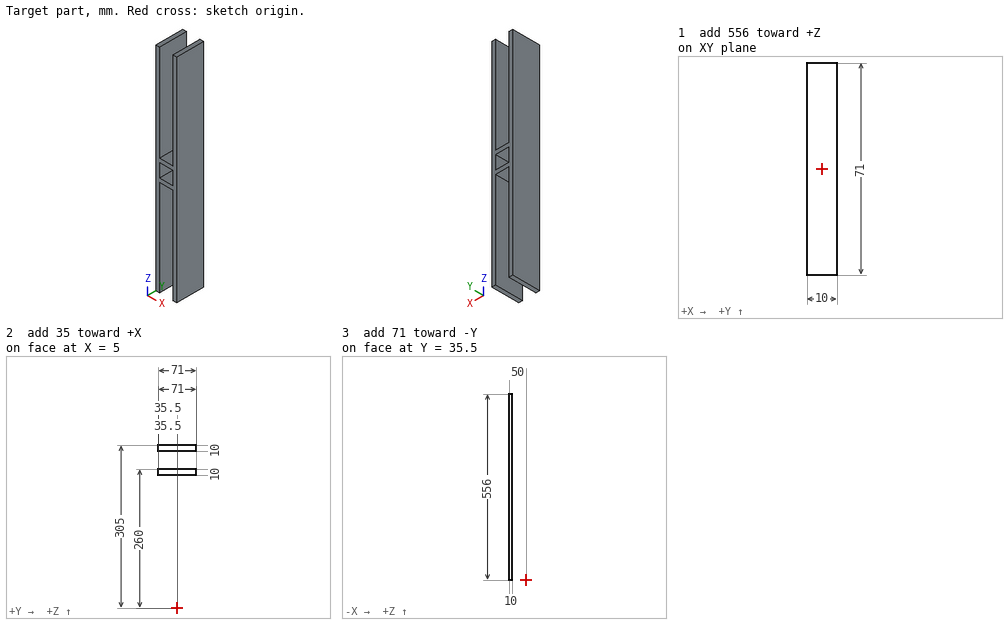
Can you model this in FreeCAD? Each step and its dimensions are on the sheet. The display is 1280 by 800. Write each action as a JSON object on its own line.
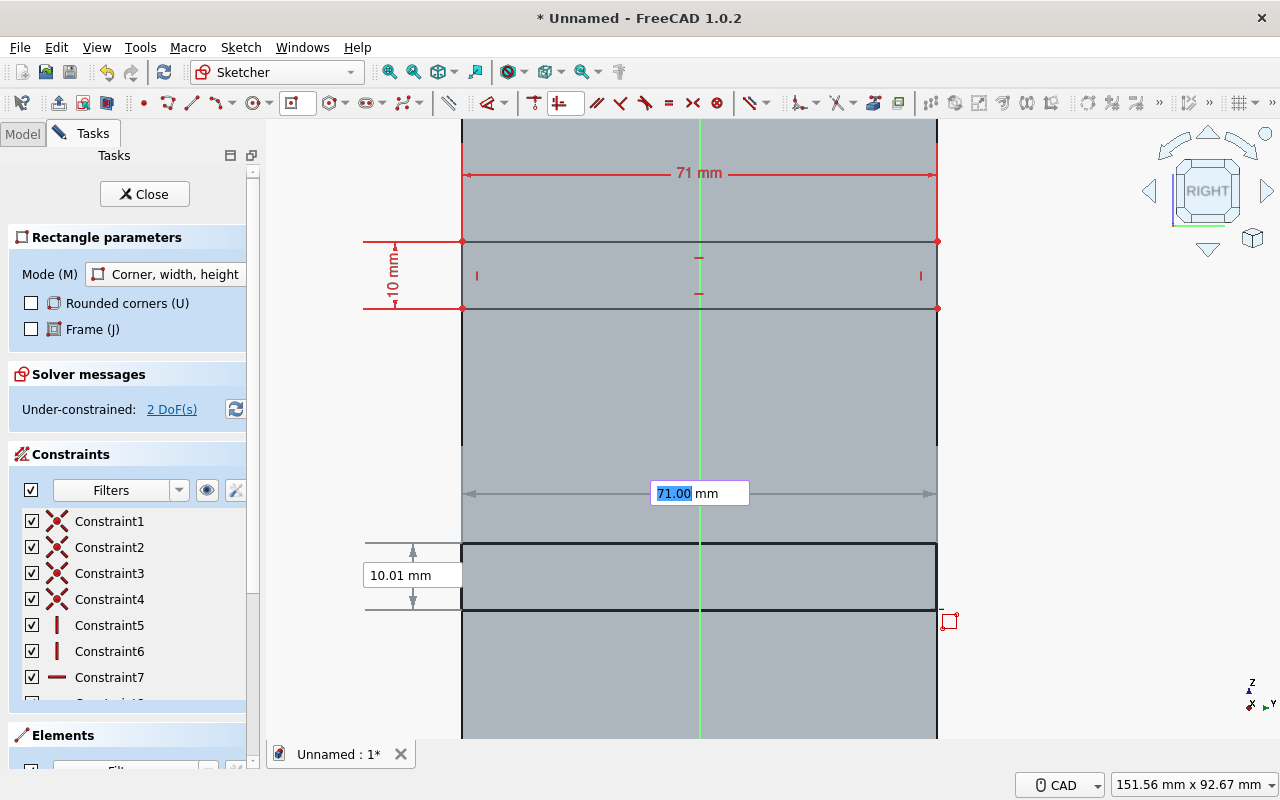
{"action": "type", "text": "71"}
{"action": "key", "text": "Tab"}
{"action": "type", "text": "10"}
{"action": "key", "text": "Return"}
{"action": "key", "text": "Escape"}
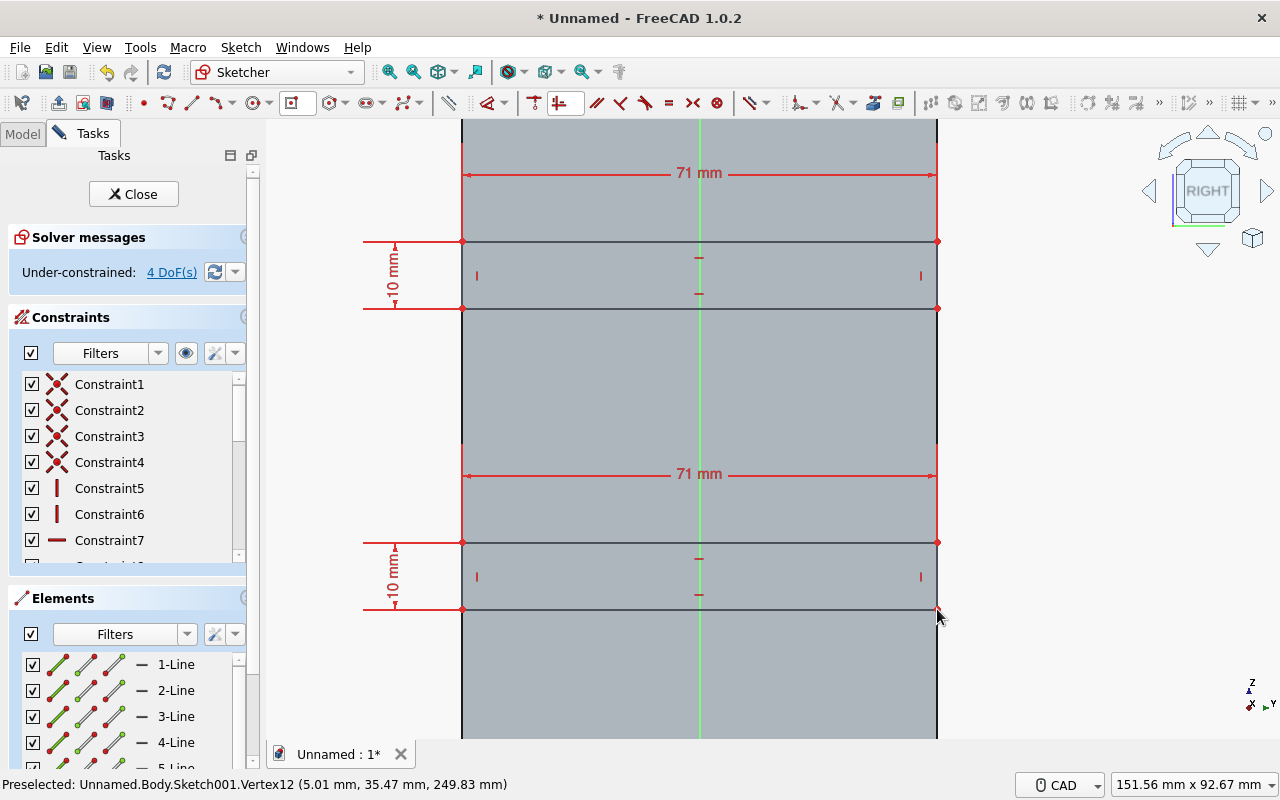
{"action": "left_click", "coordinate": [462, 242]}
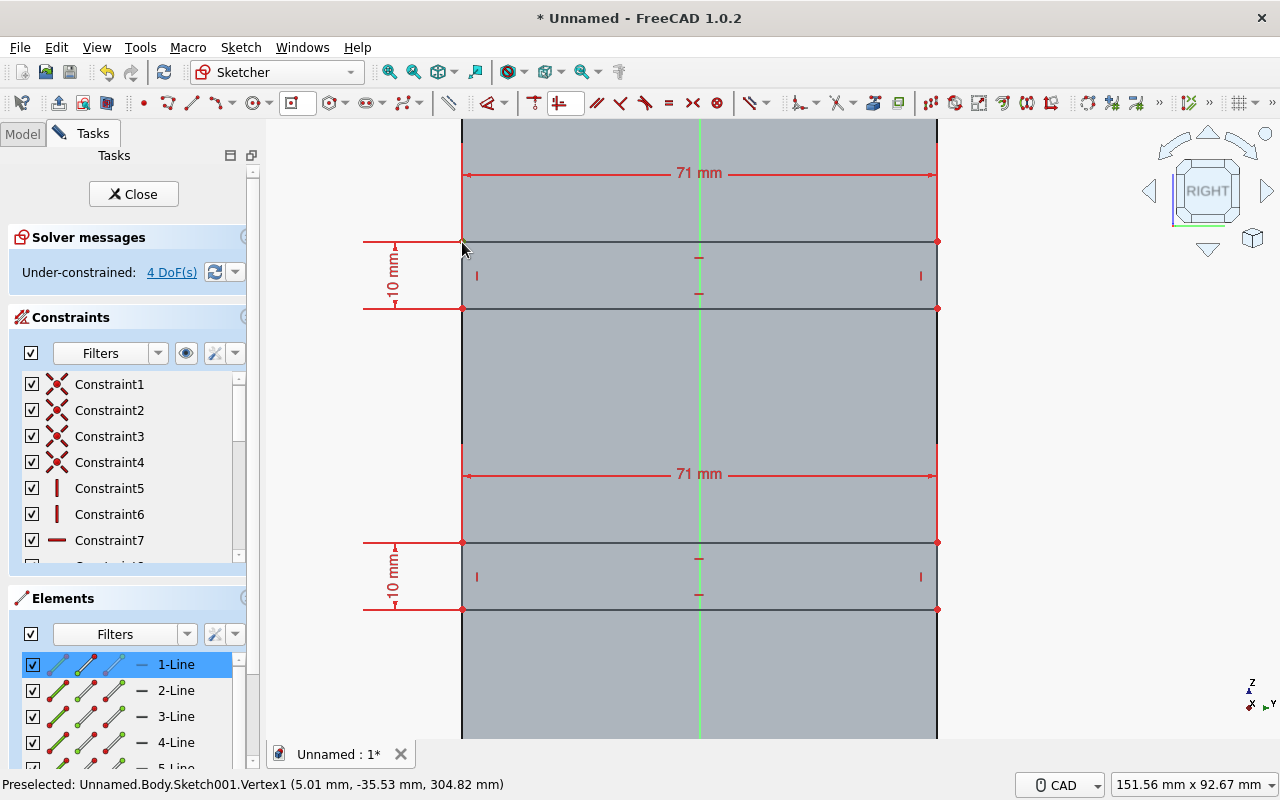
{"action": "left_click", "coordinate": [506, 104]}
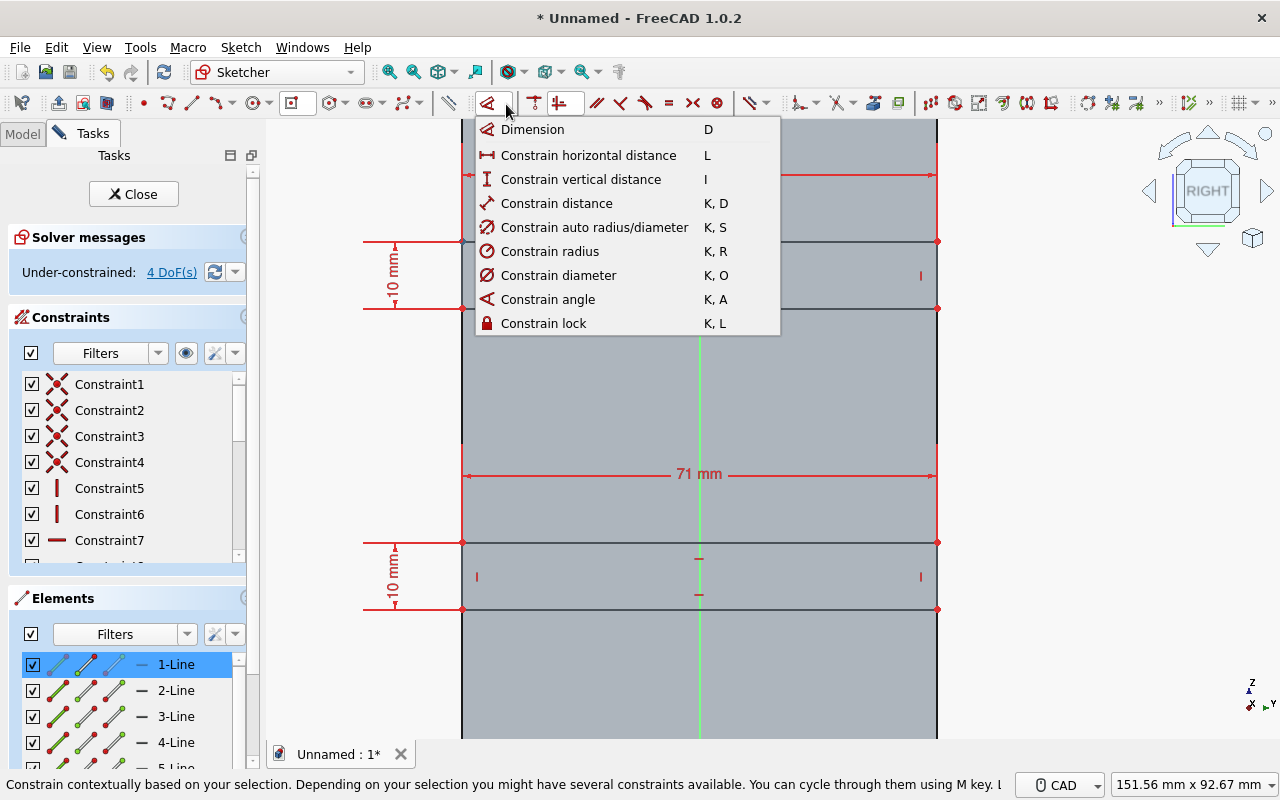
{"action": "left_click", "coordinate": [628, 179]}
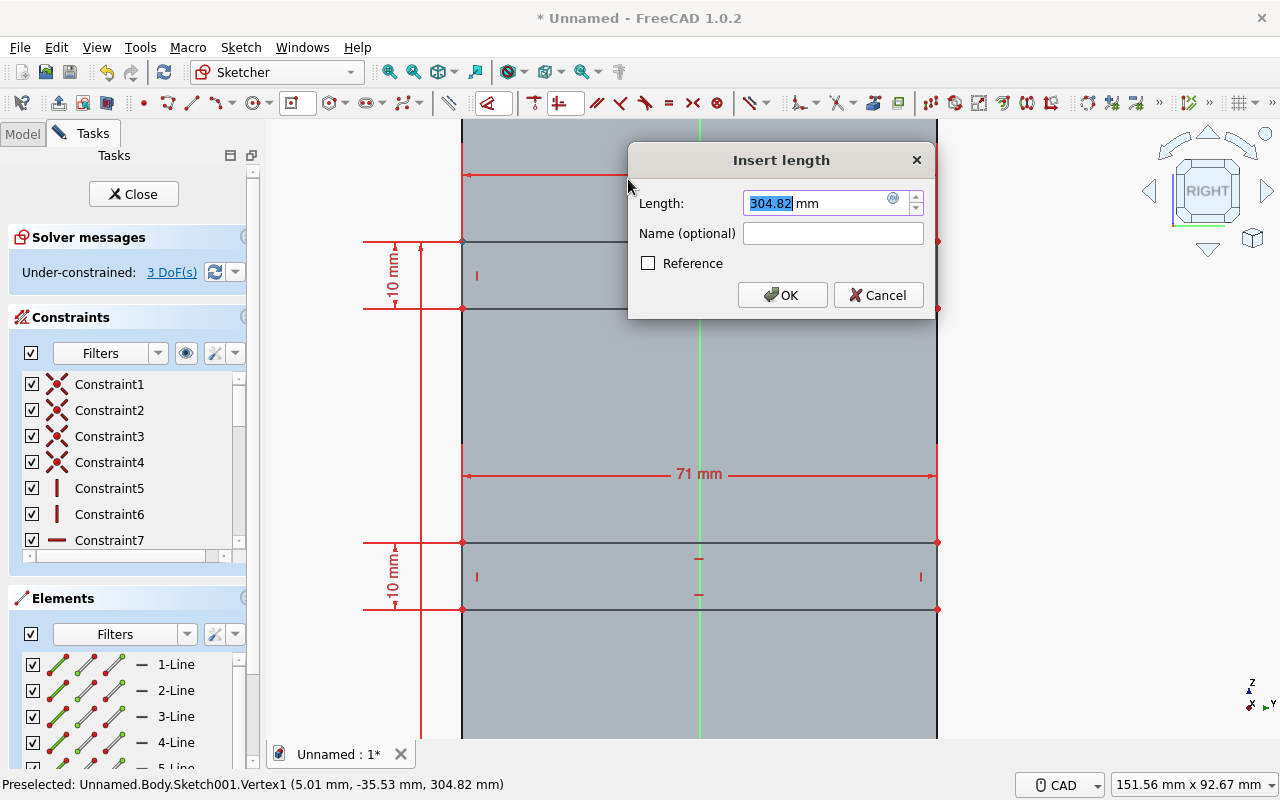
{"action": "type", "text": "305"}
{"action": "key", "text": "Return"}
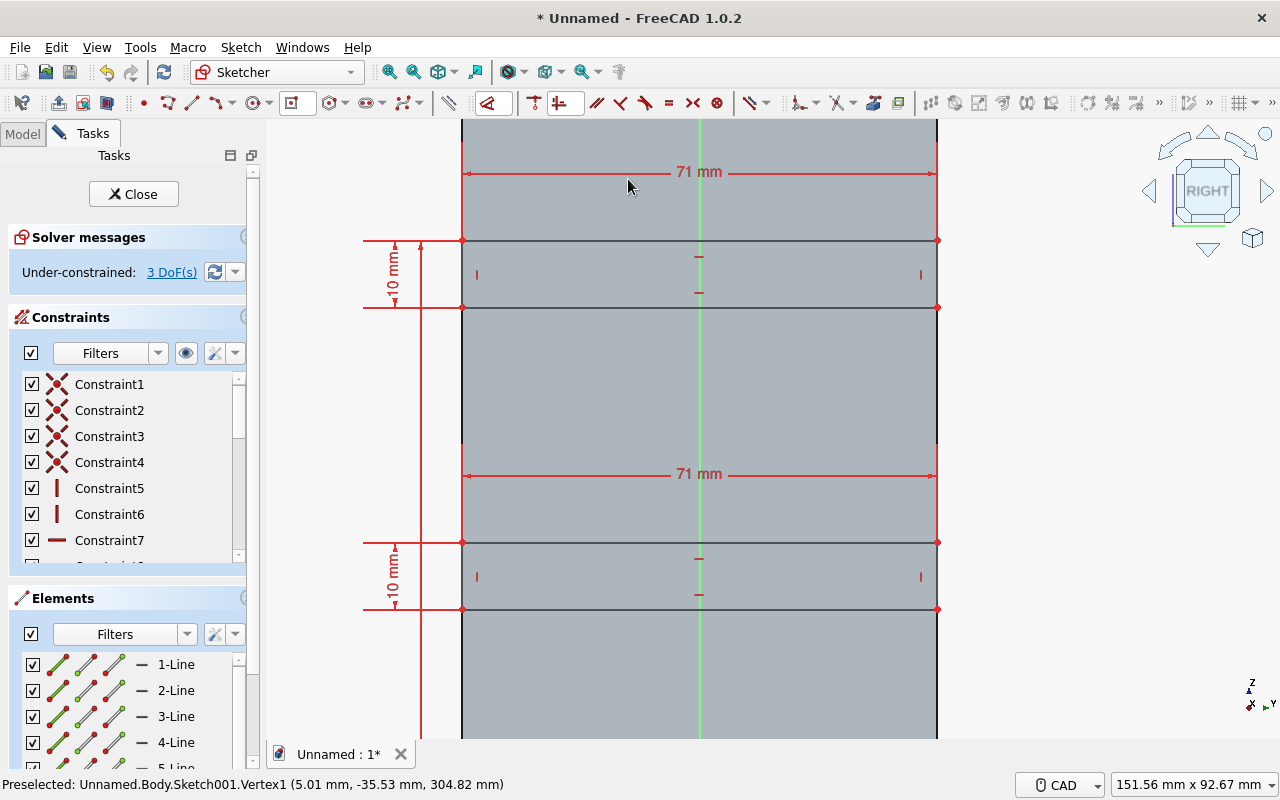
{"action": "left_click", "coordinate": [462, 543]}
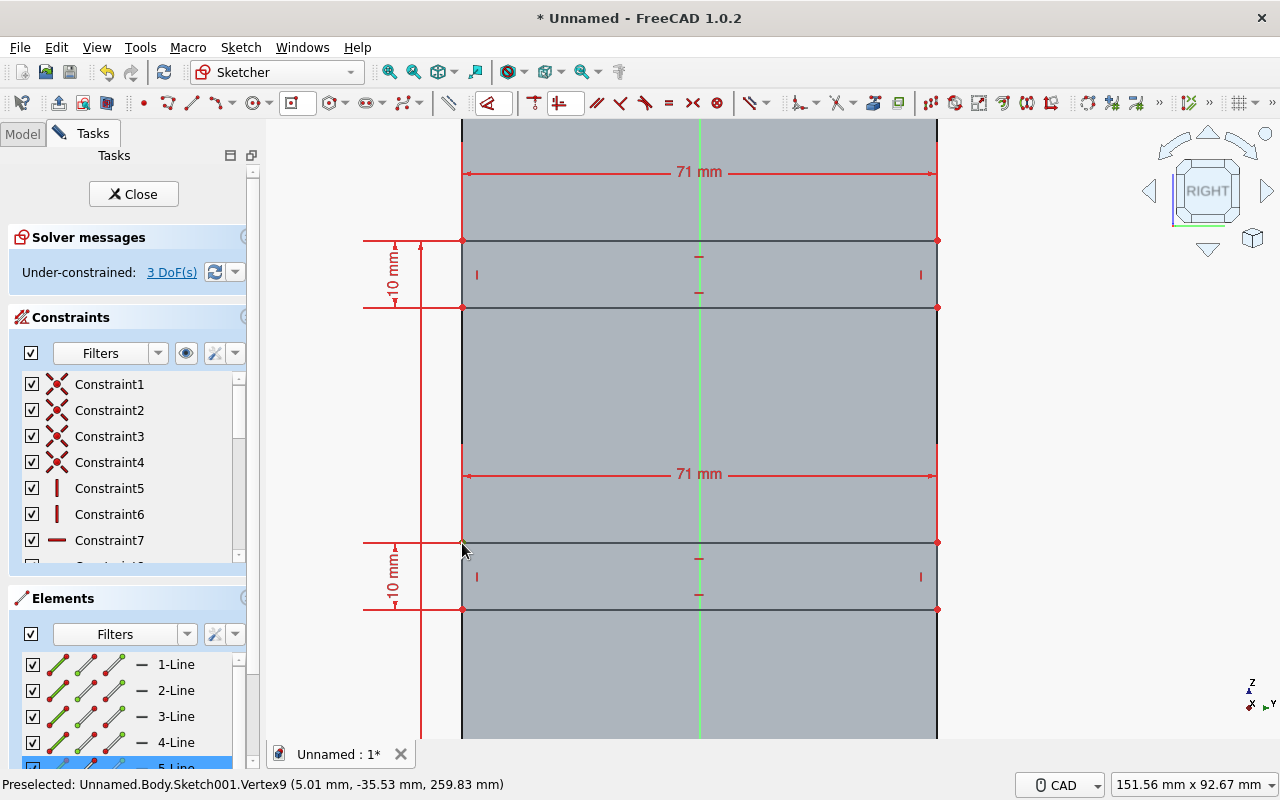
{"action": "left_click", "coordinate": [506, 104]}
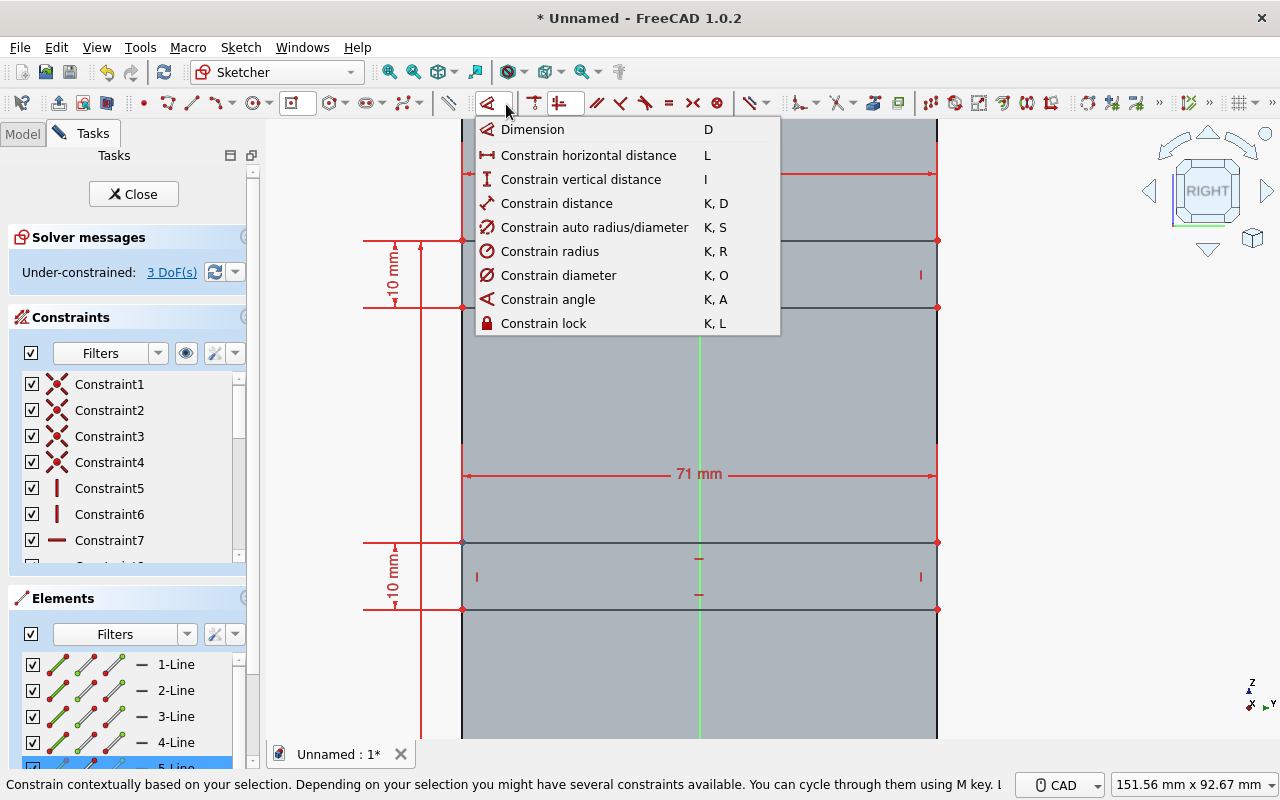
{"action": "left_click", "coordinate": [628, 179]}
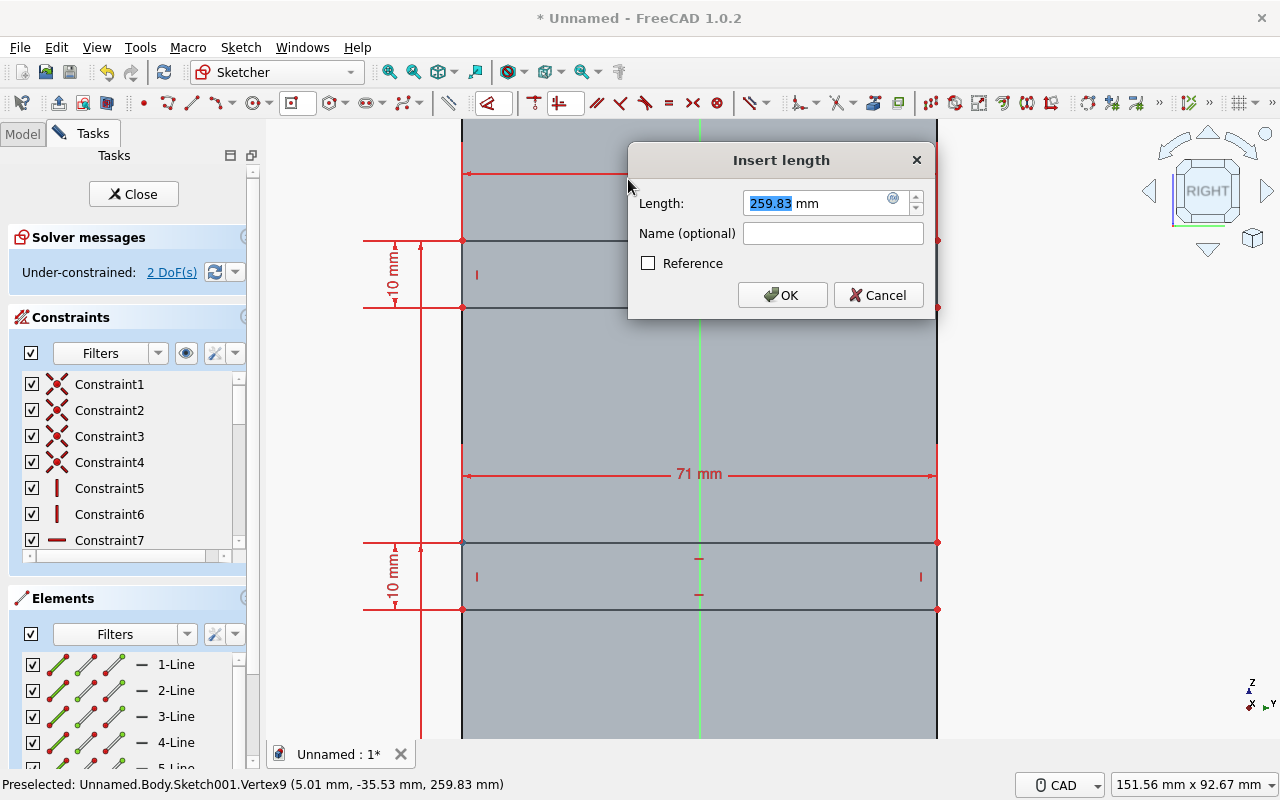
{"action": "type", "text": "260"}
{"action": "key", "text": "Return"}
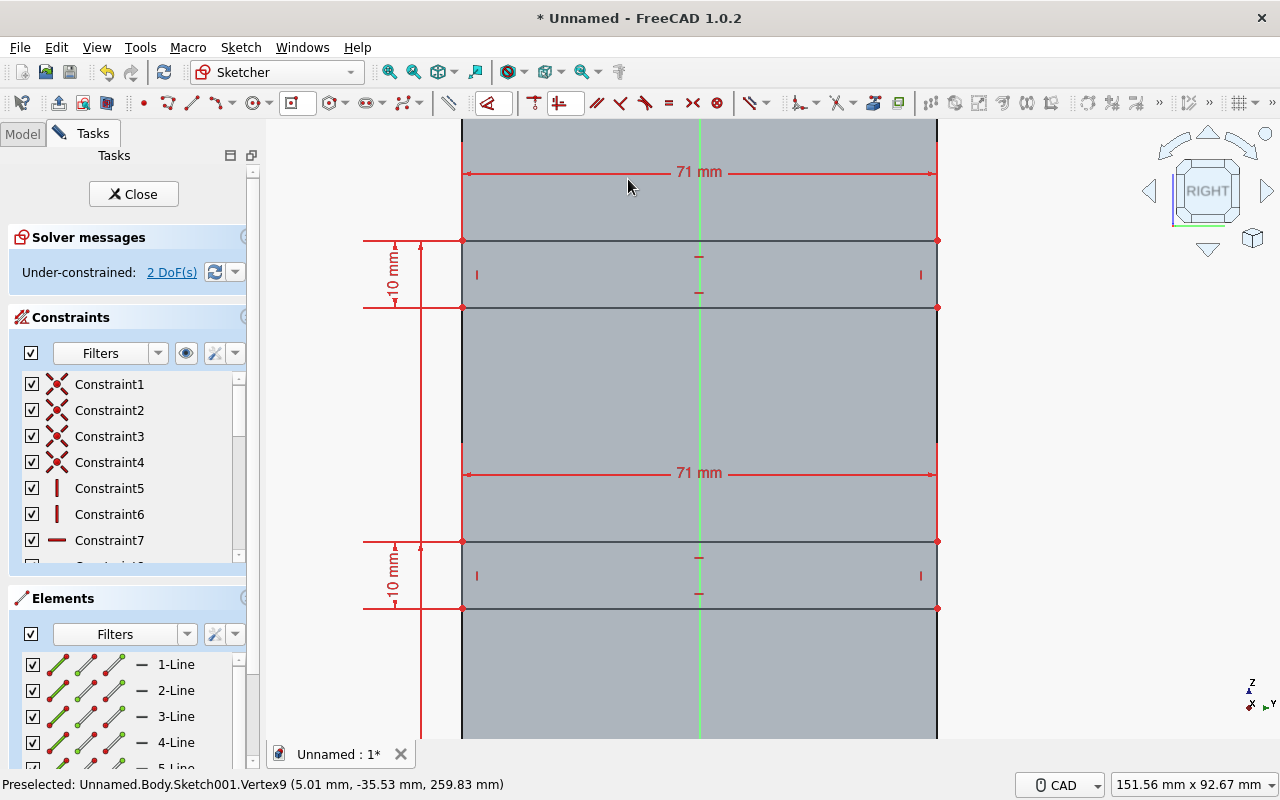
{"action": "left_click", "coordinate": [462, 241]}